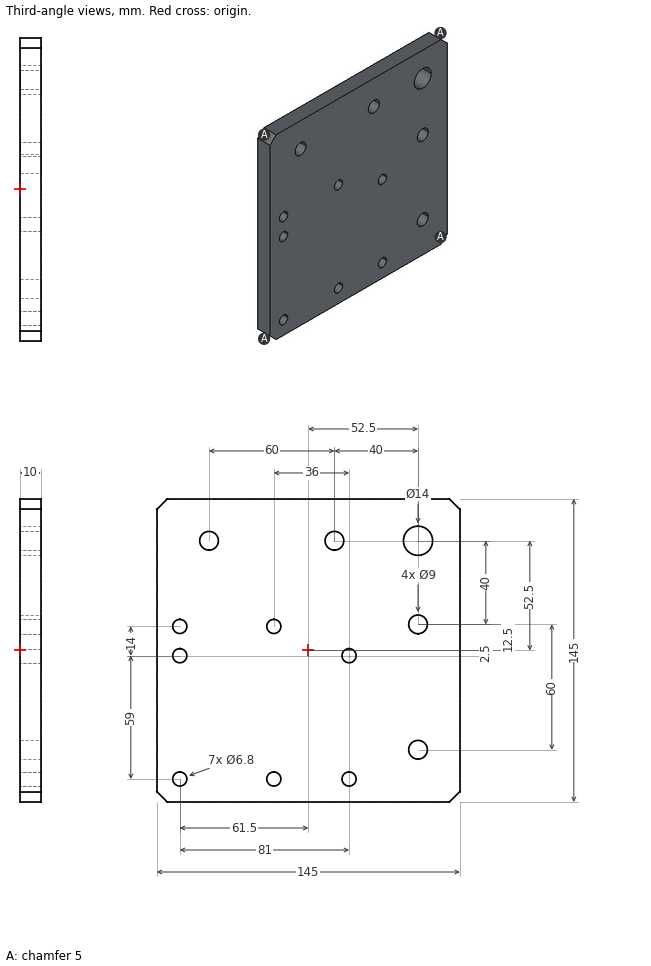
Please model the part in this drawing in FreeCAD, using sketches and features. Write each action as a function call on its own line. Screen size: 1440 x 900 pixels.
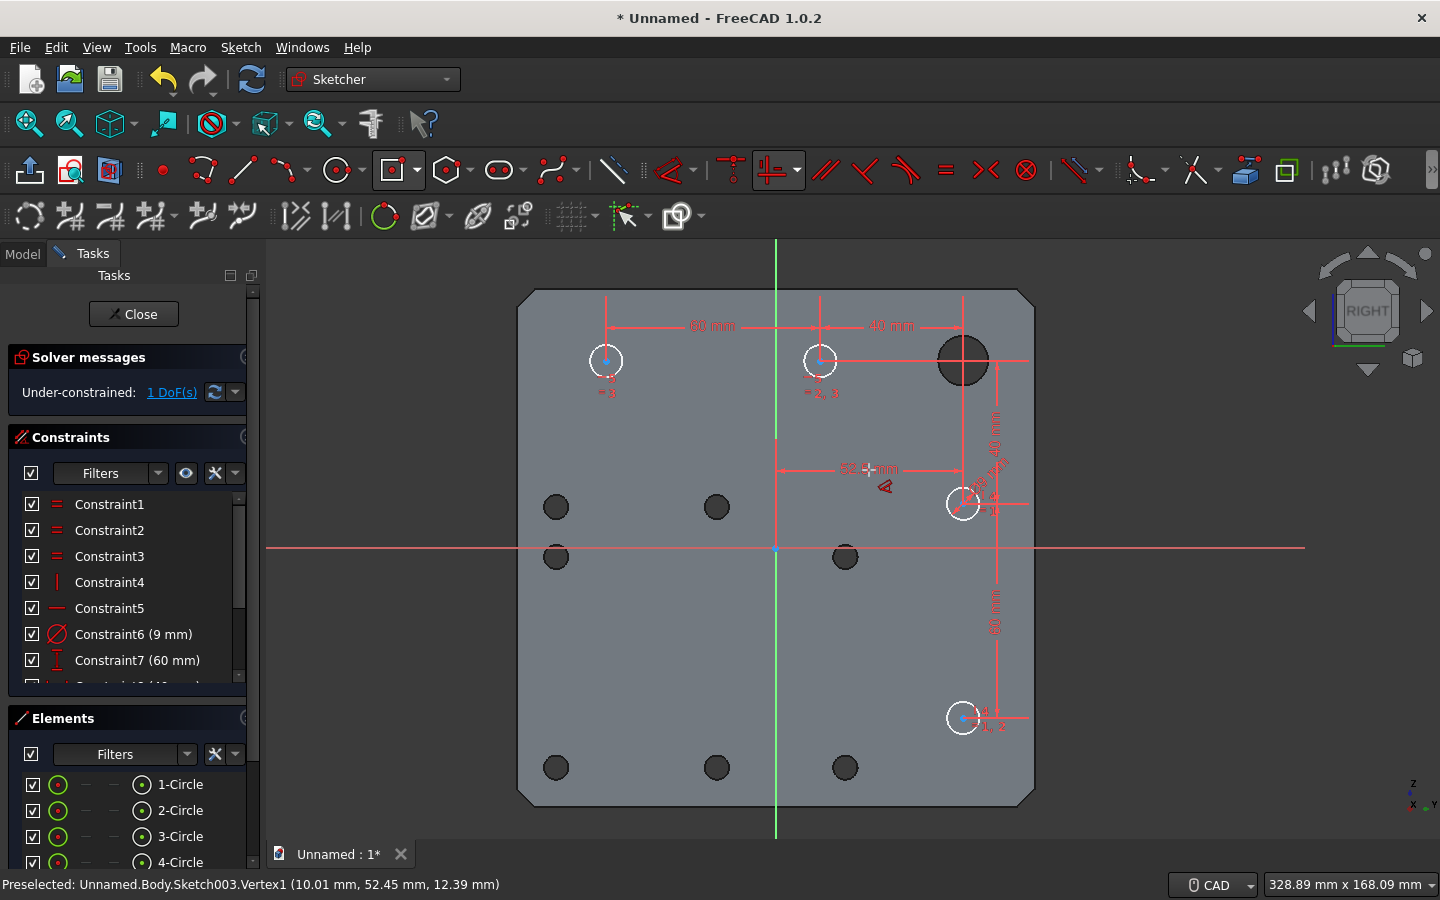
click(963, 504)
click(997, 526)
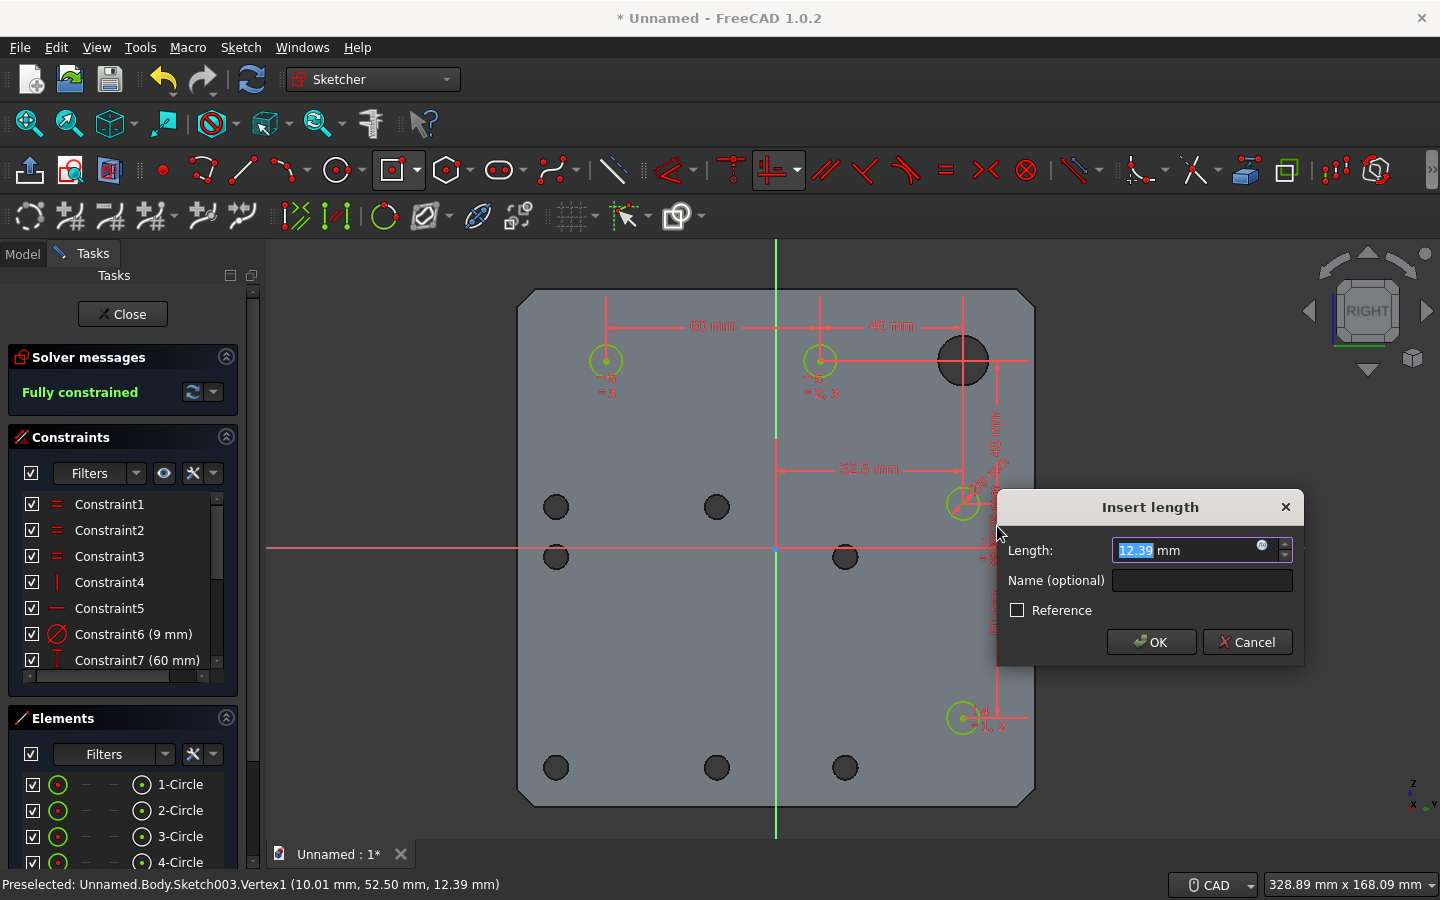
text(12.5)
key(Return)
key(Escape)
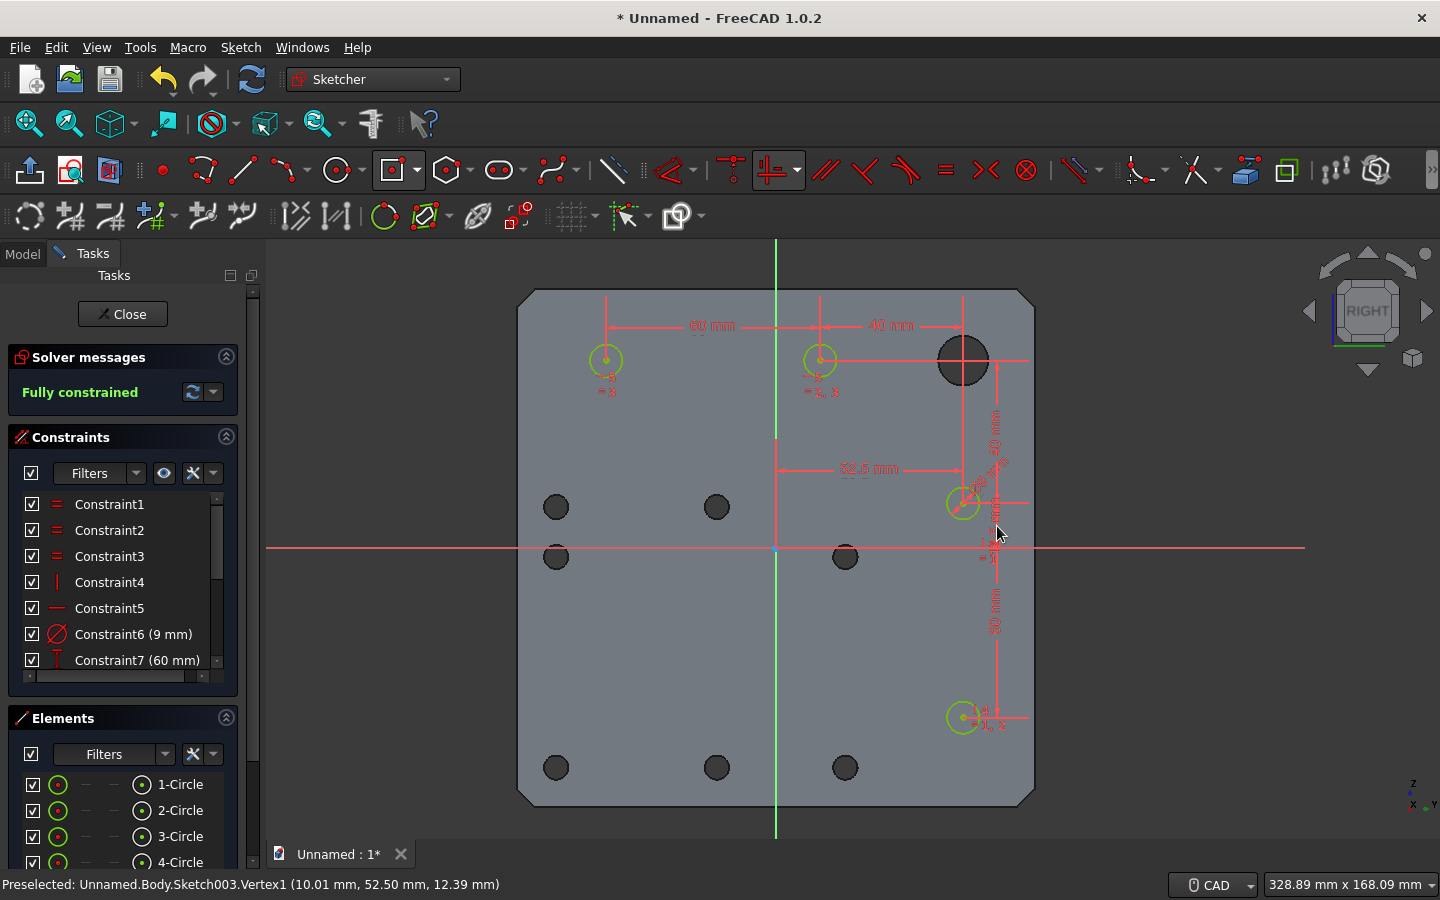
click(123, 314)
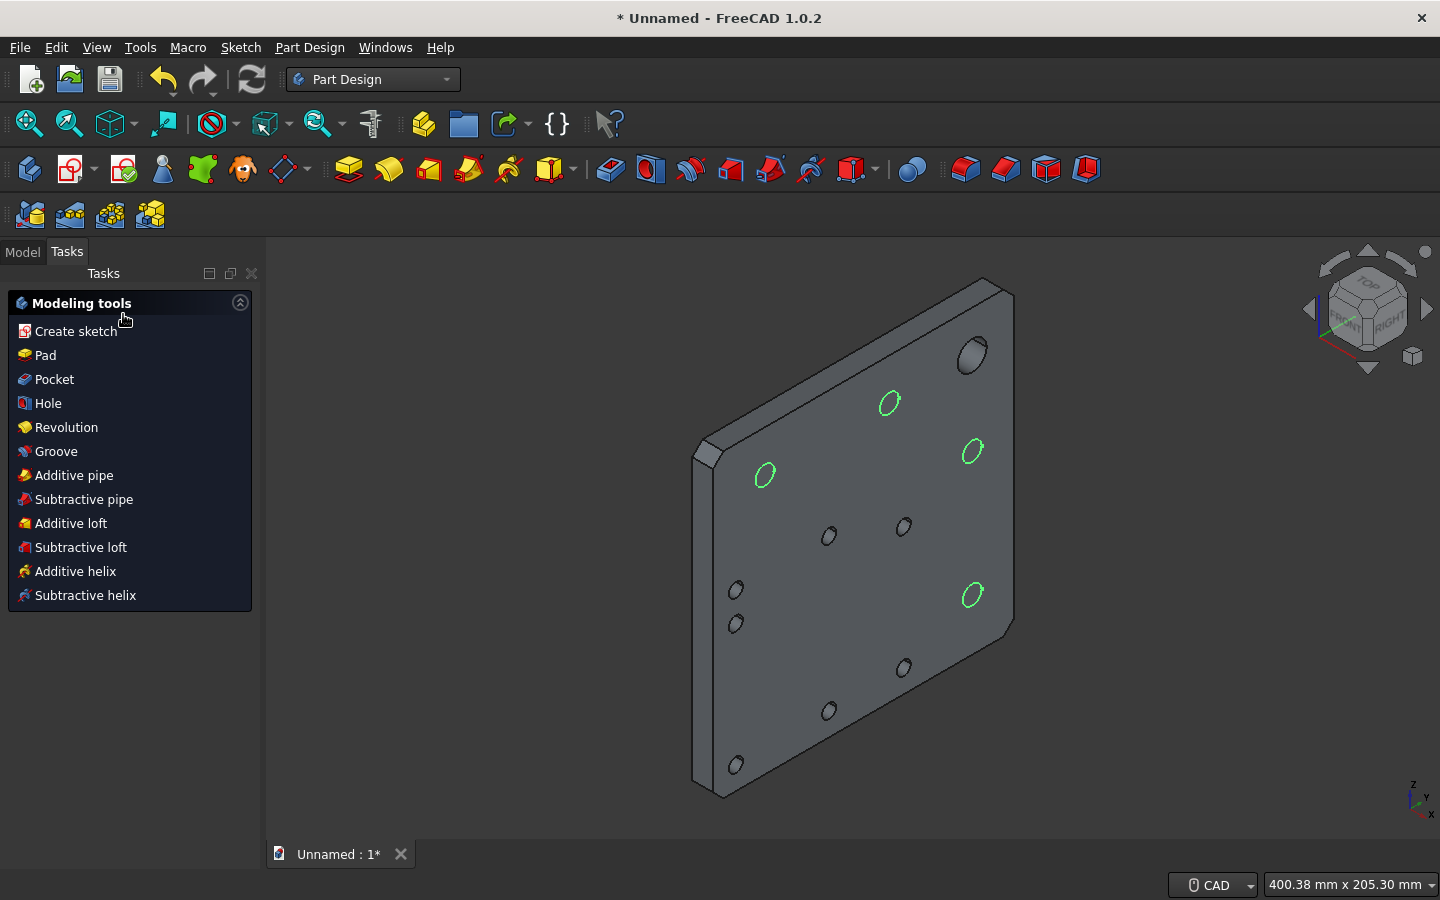
click(612, 170)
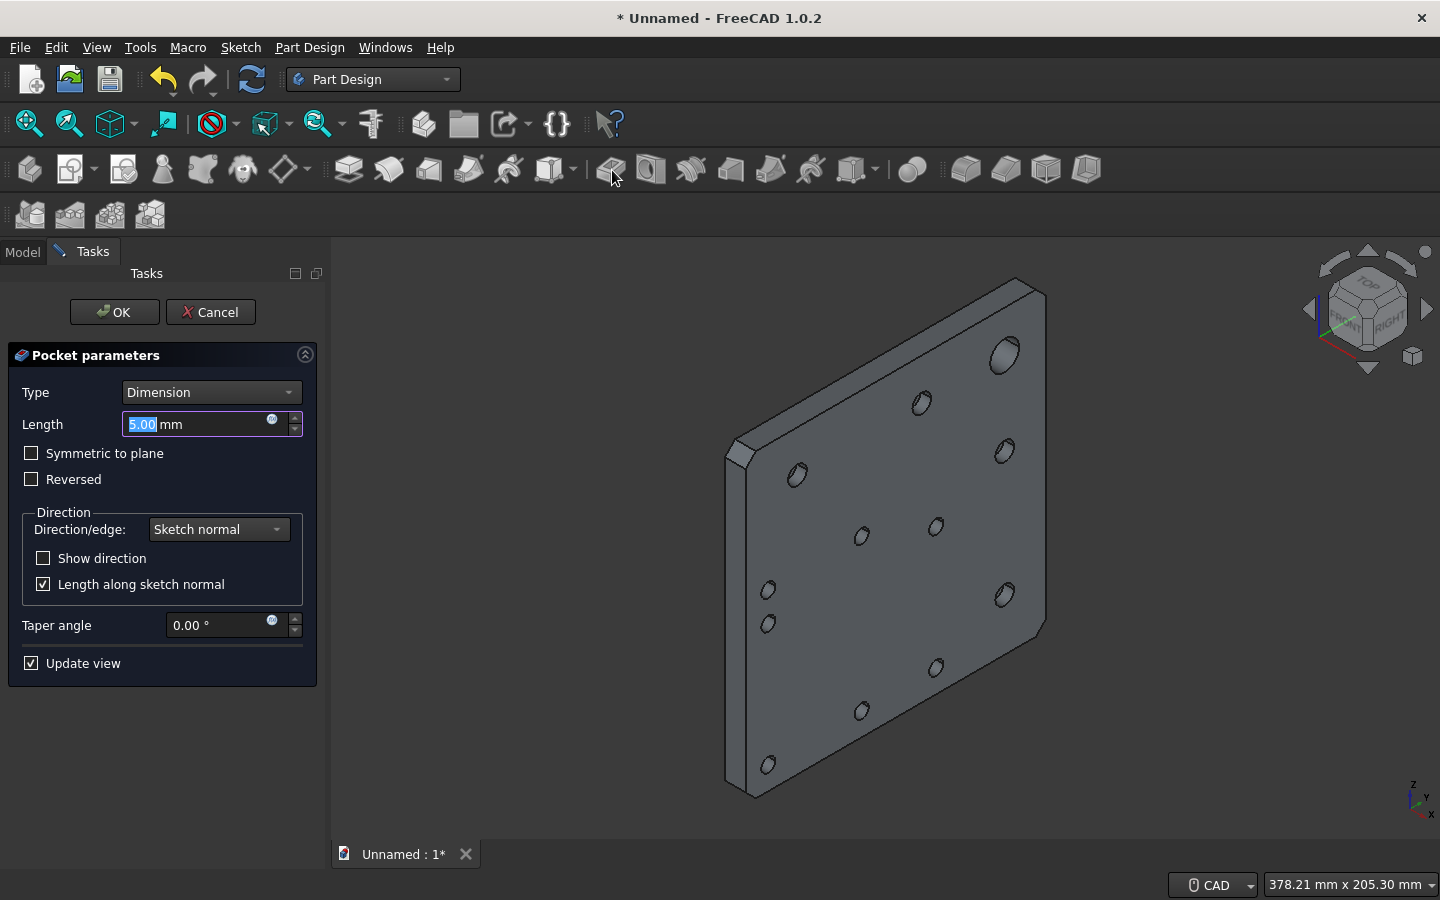
click(212, 392)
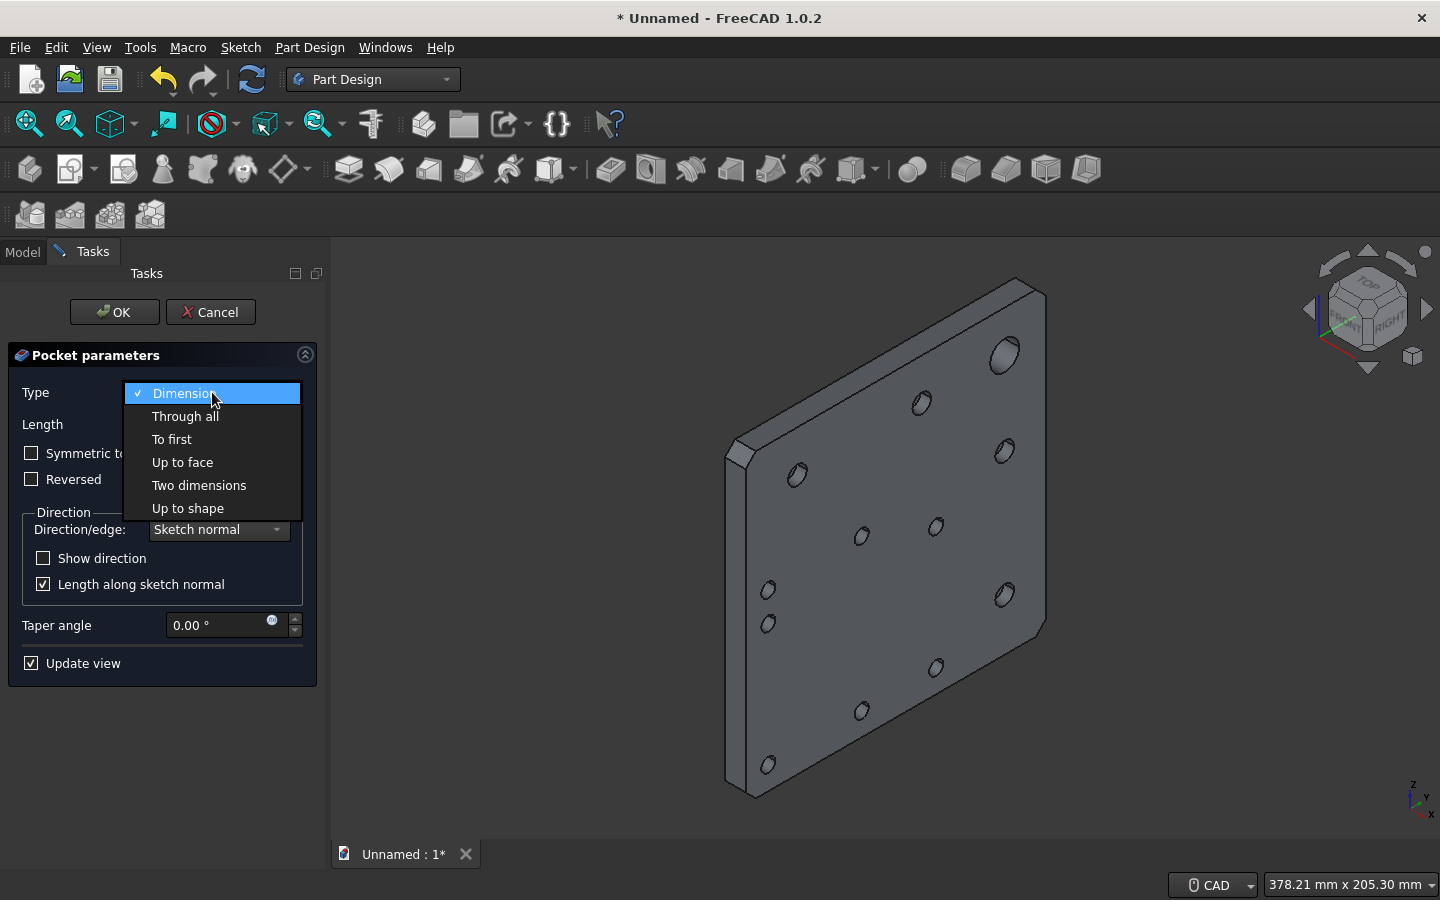
click(212, 416)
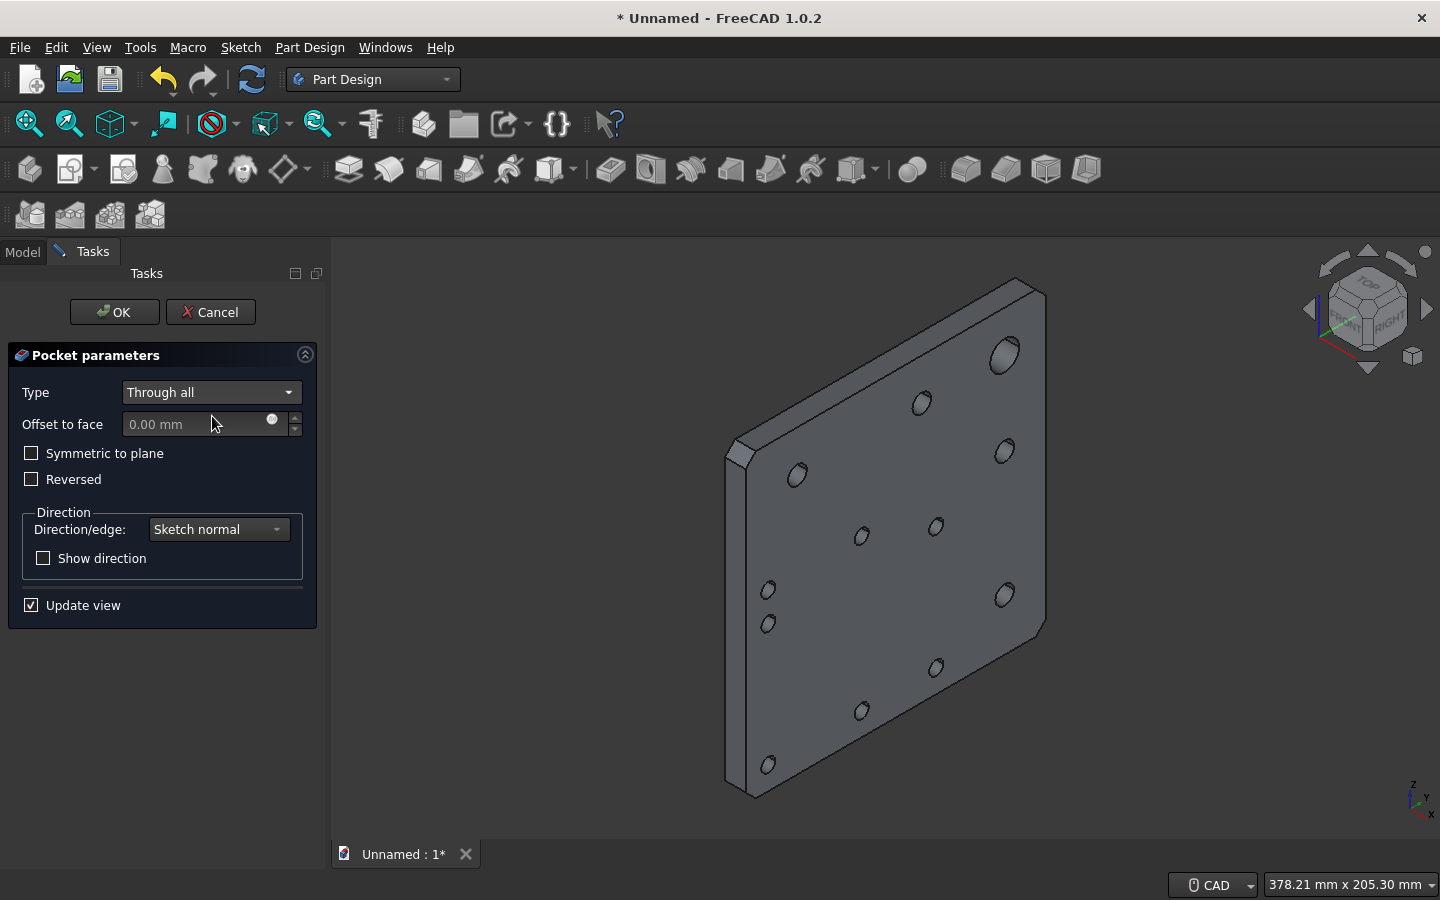
click(115, 312)